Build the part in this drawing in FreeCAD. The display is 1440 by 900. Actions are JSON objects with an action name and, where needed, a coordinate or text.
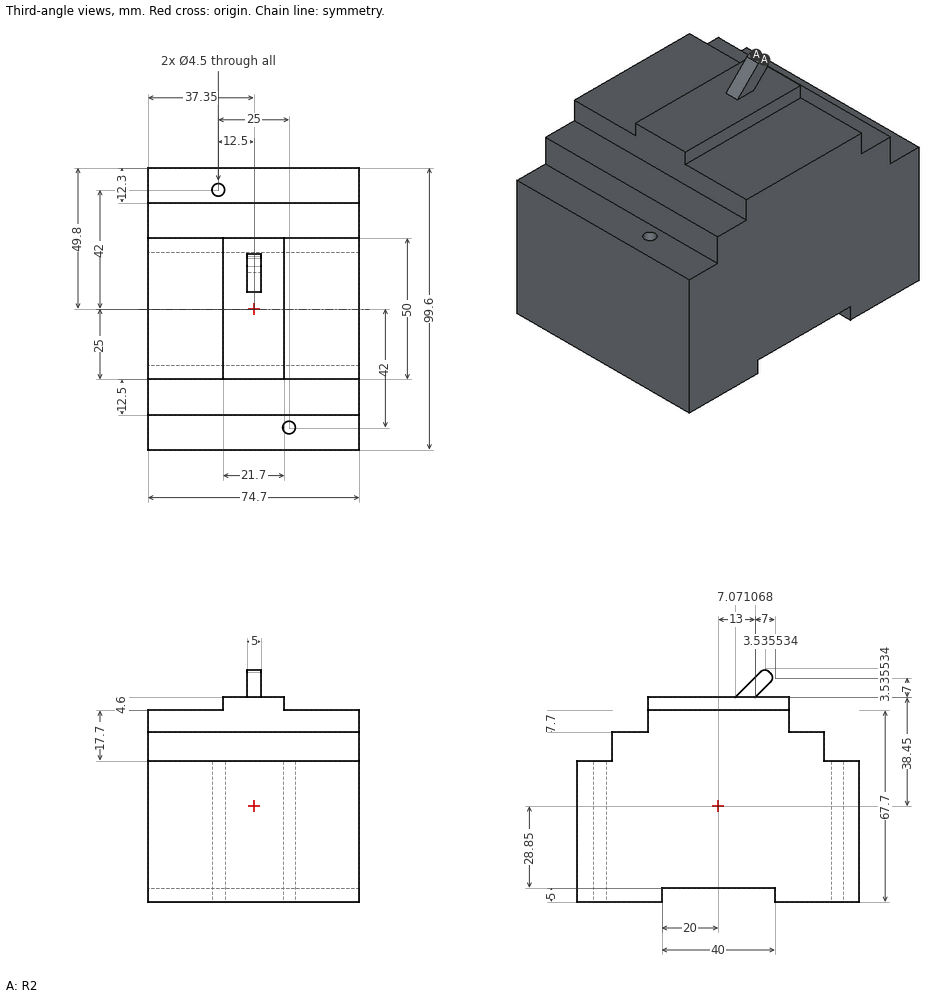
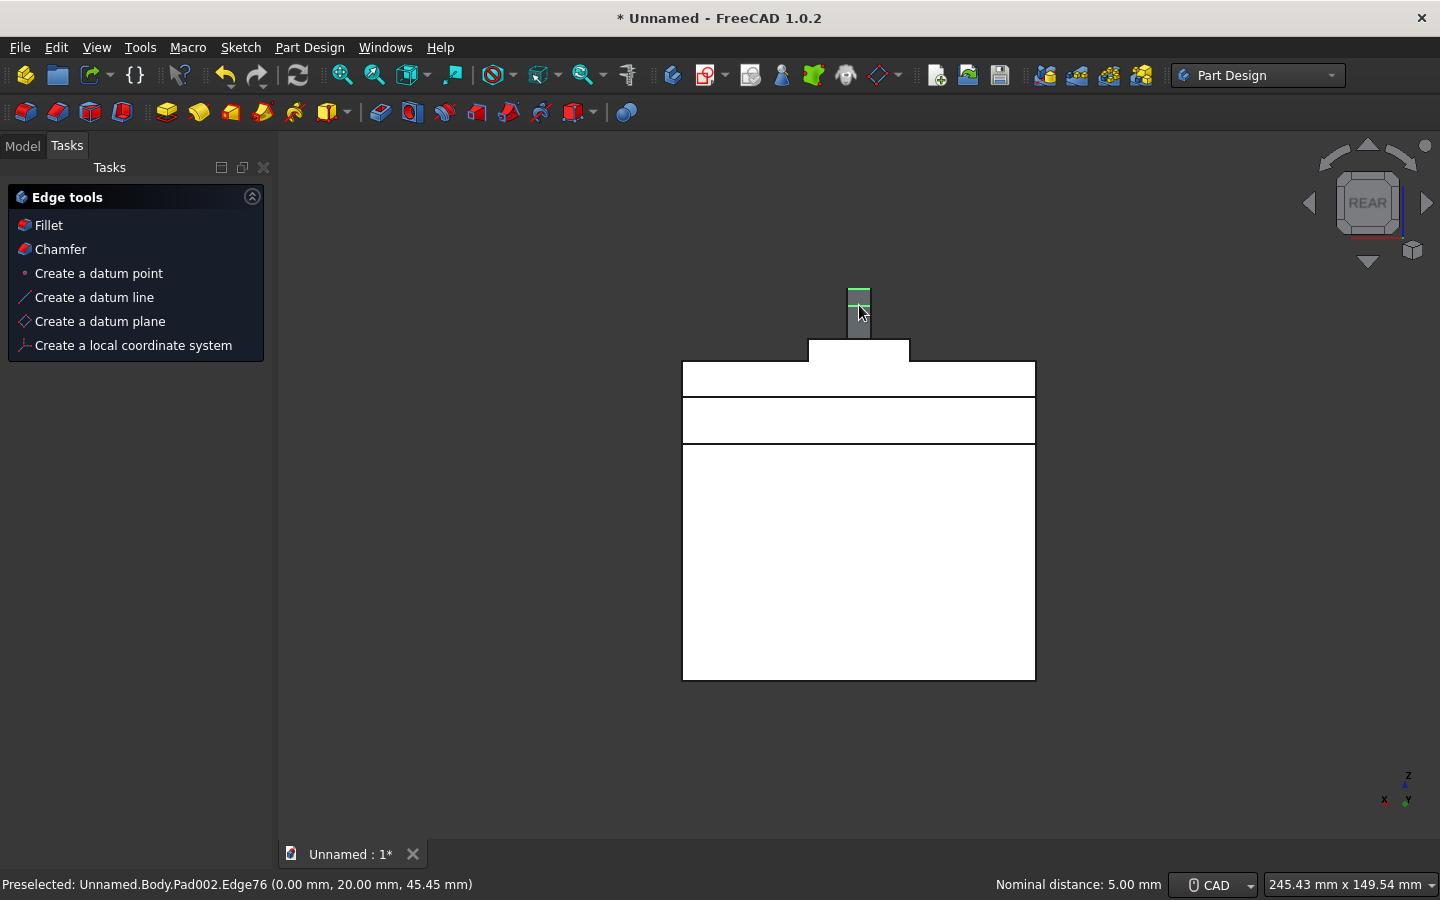
{"action": "left_click", "coordinate": [26, 112]}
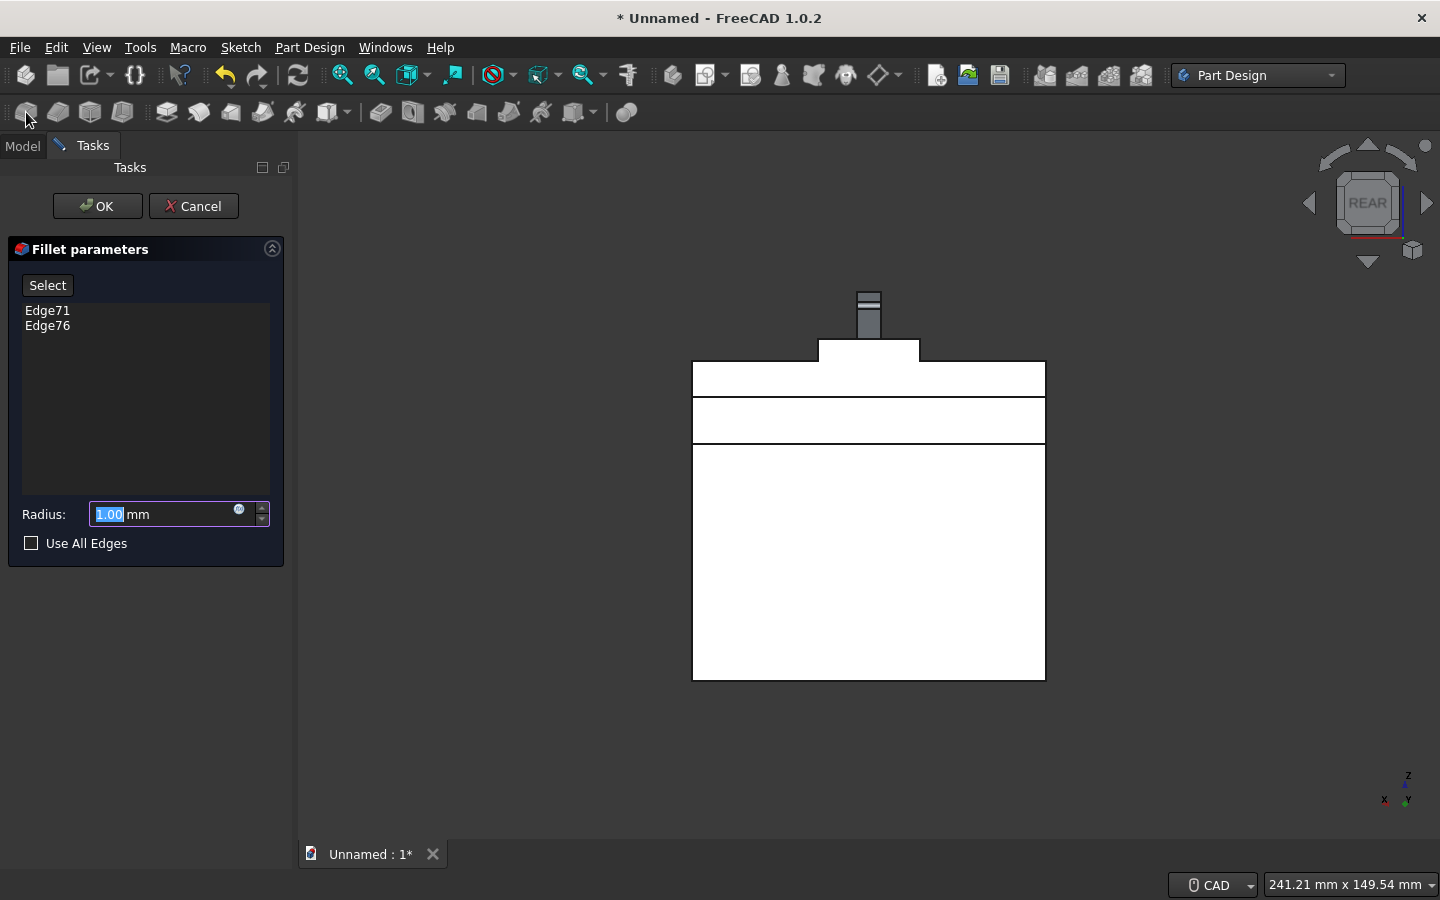
{"action": "type", "text": "2"}
{"action": "key", "text": "Tab"}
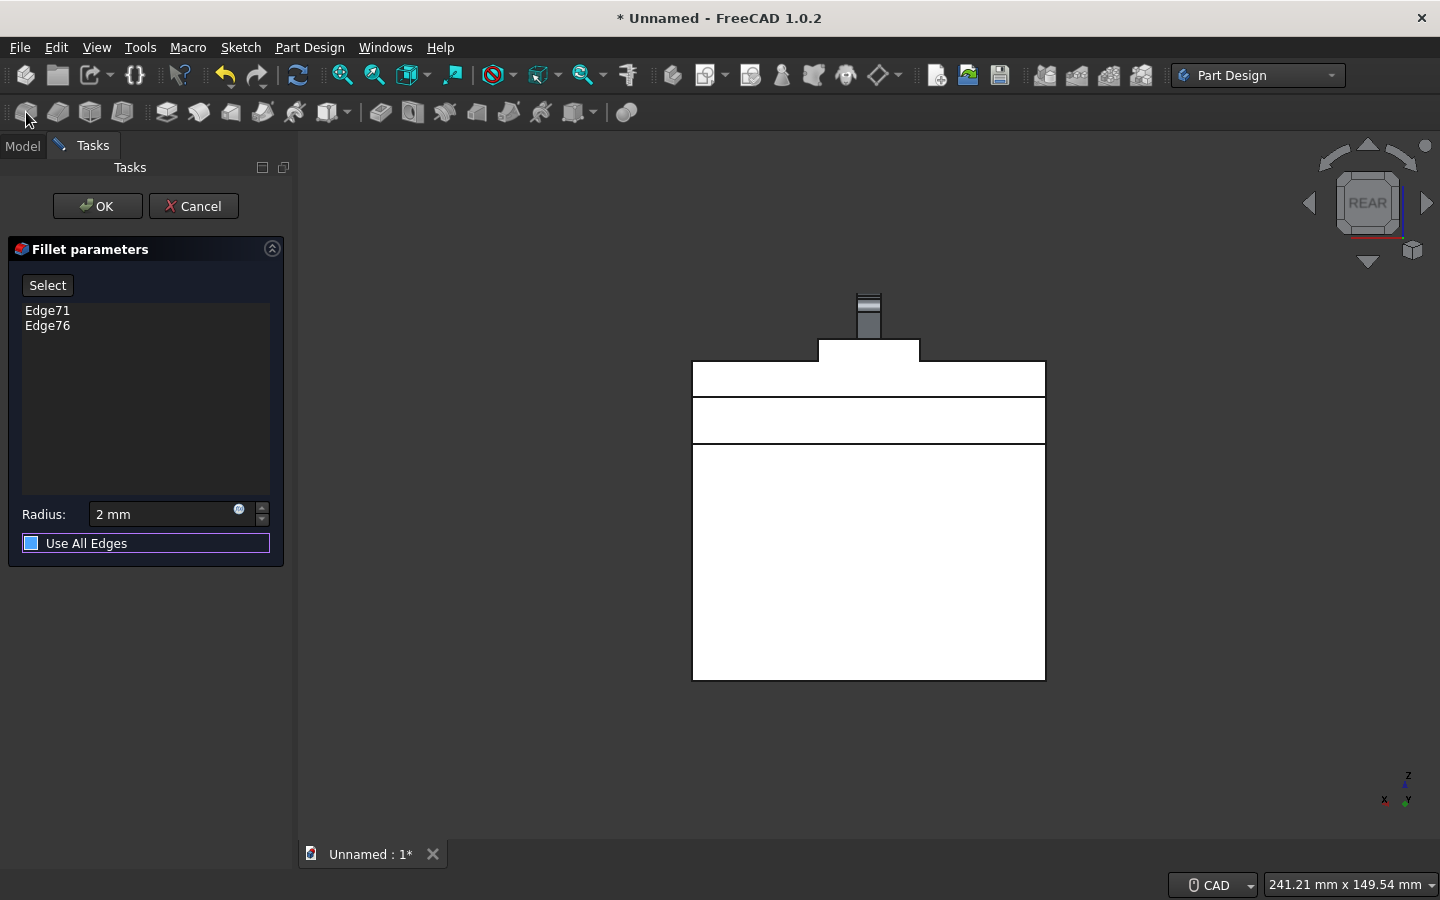
{"action": "left_click", "coordinate": [98, 206]}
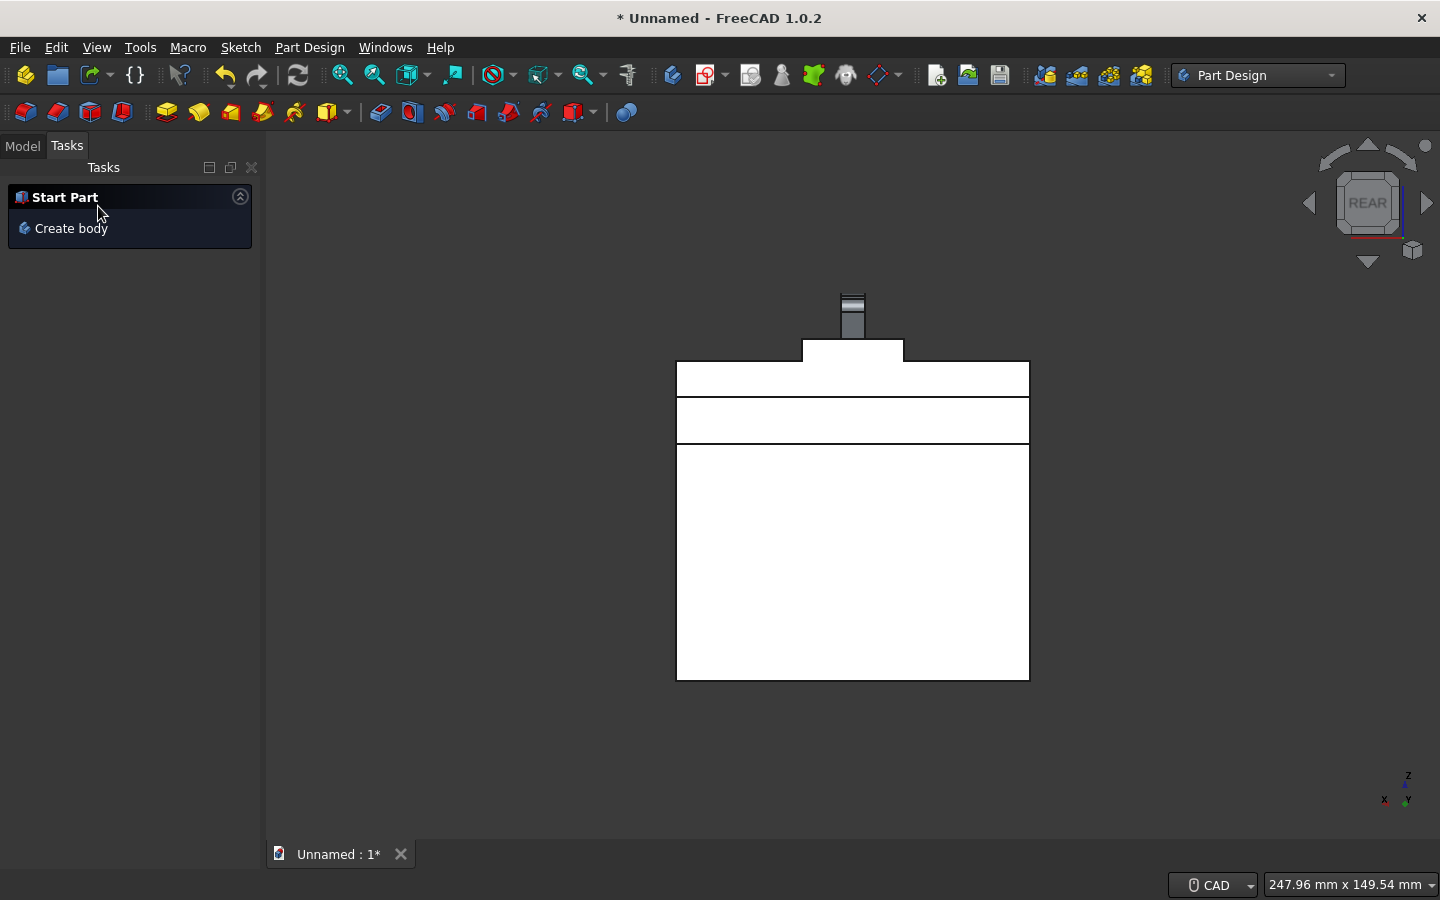
{"action": "key", "text": "0"}